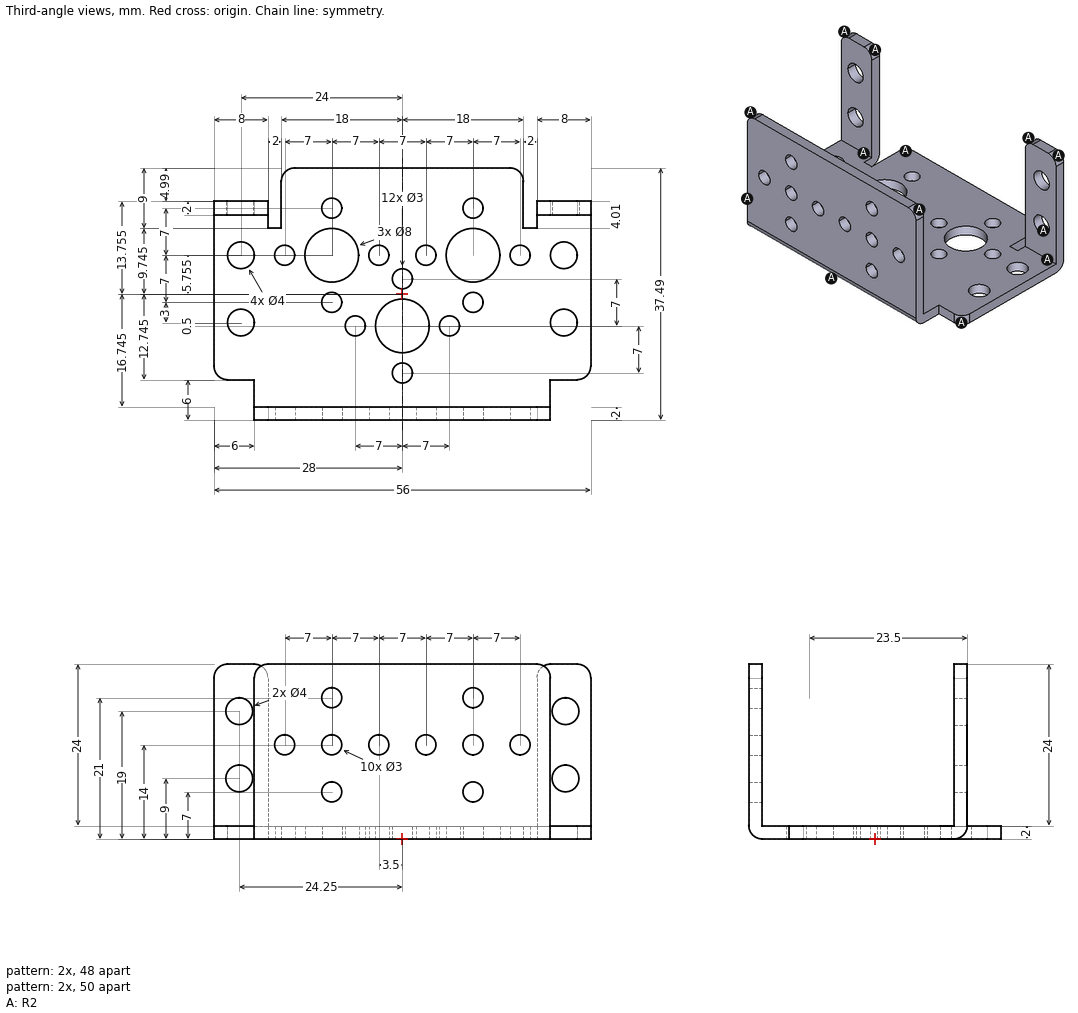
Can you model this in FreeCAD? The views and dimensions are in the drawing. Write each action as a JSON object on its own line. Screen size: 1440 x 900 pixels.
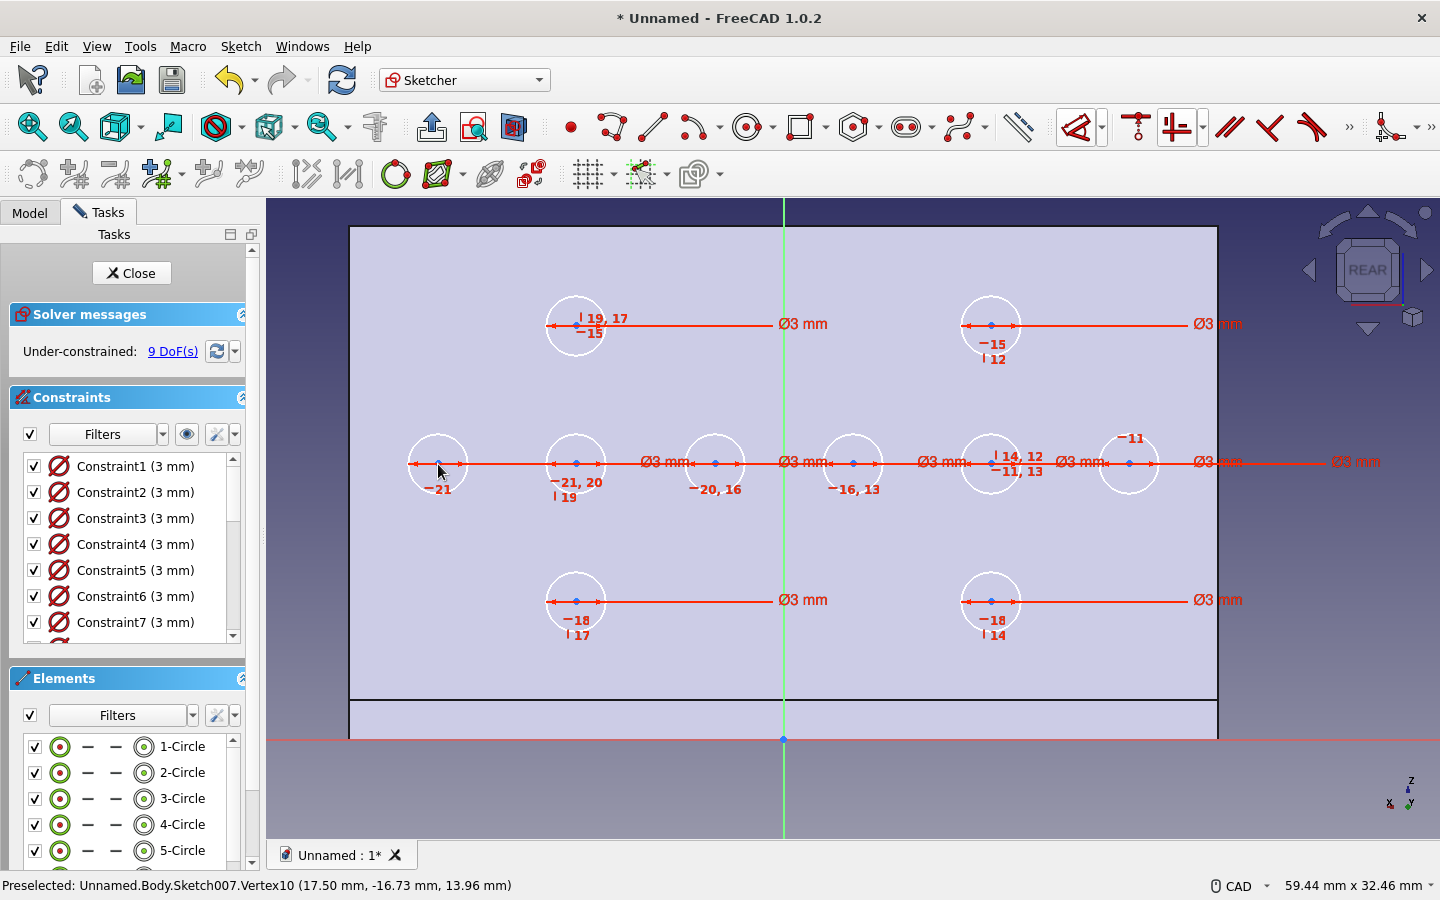
{"action": "left_click", "coordinate": [991, 602]}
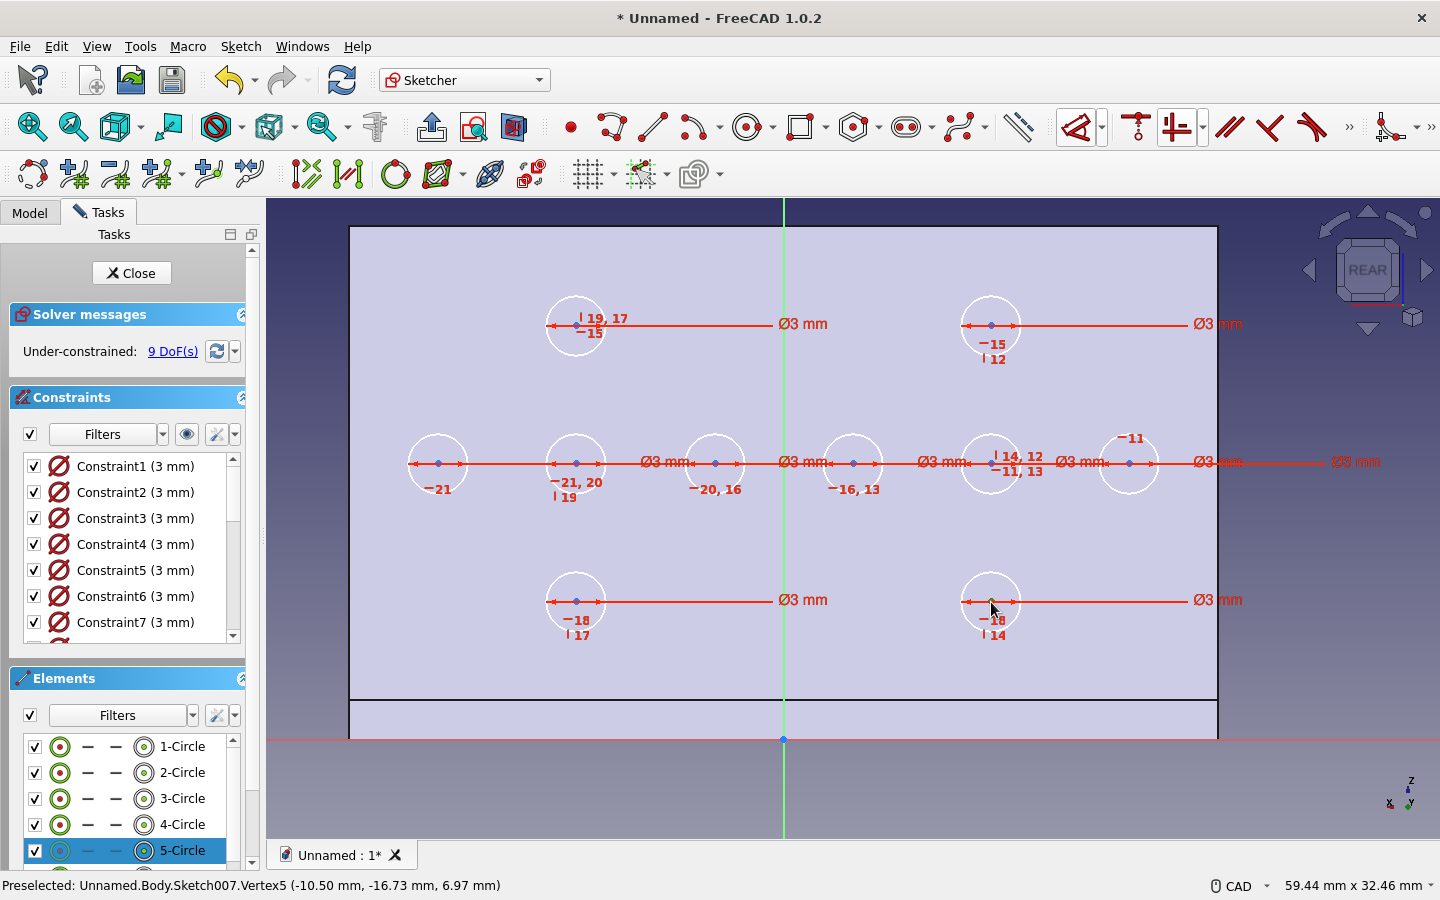
{"action": "key", "text": "i"}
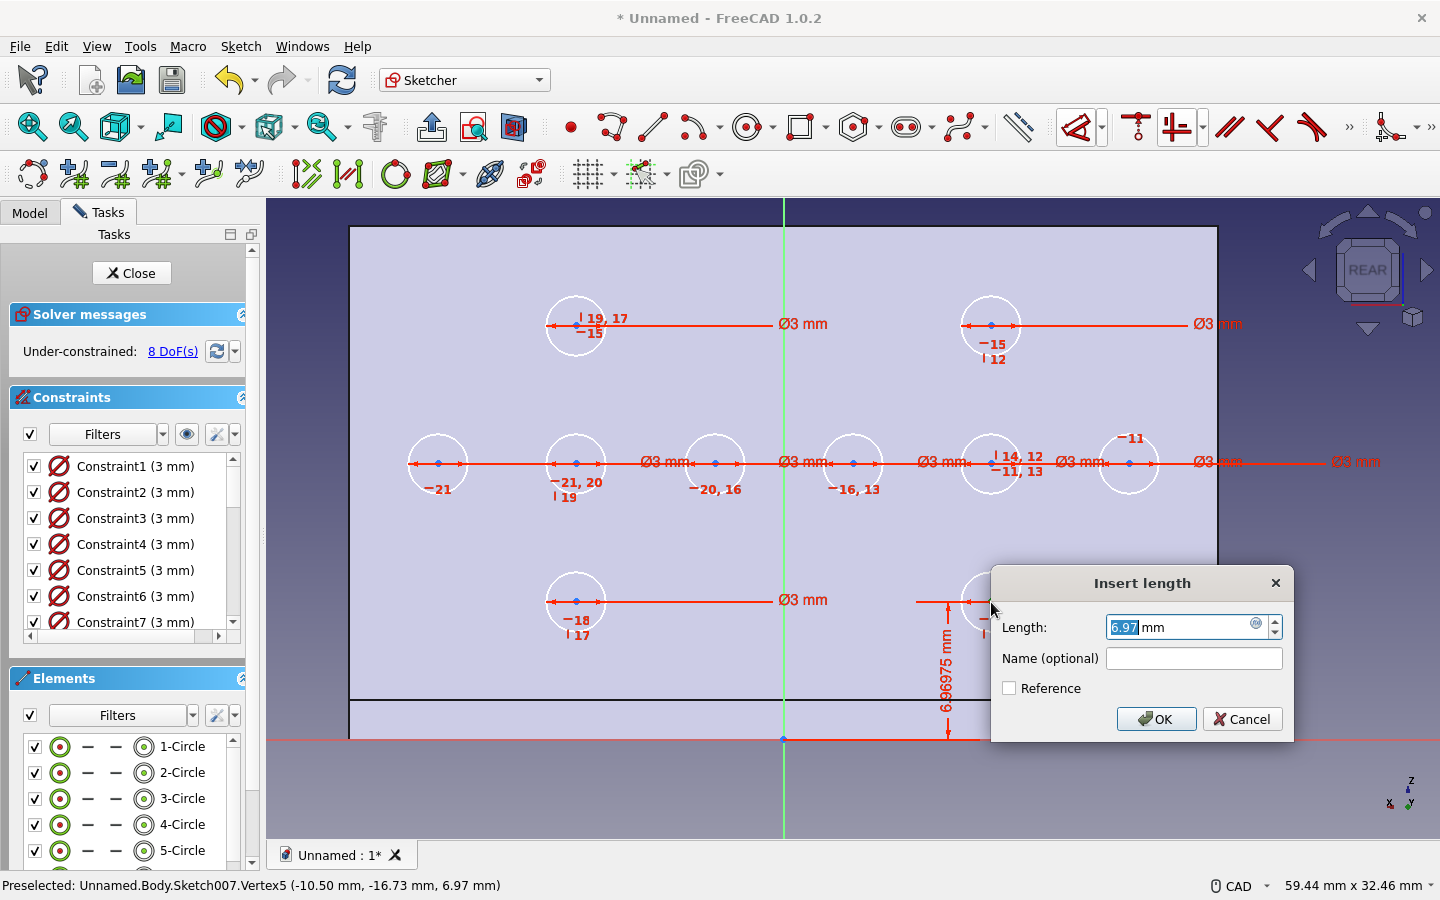
{"action": "type", "text": "7"}
{"action": "key", "text": "Return"}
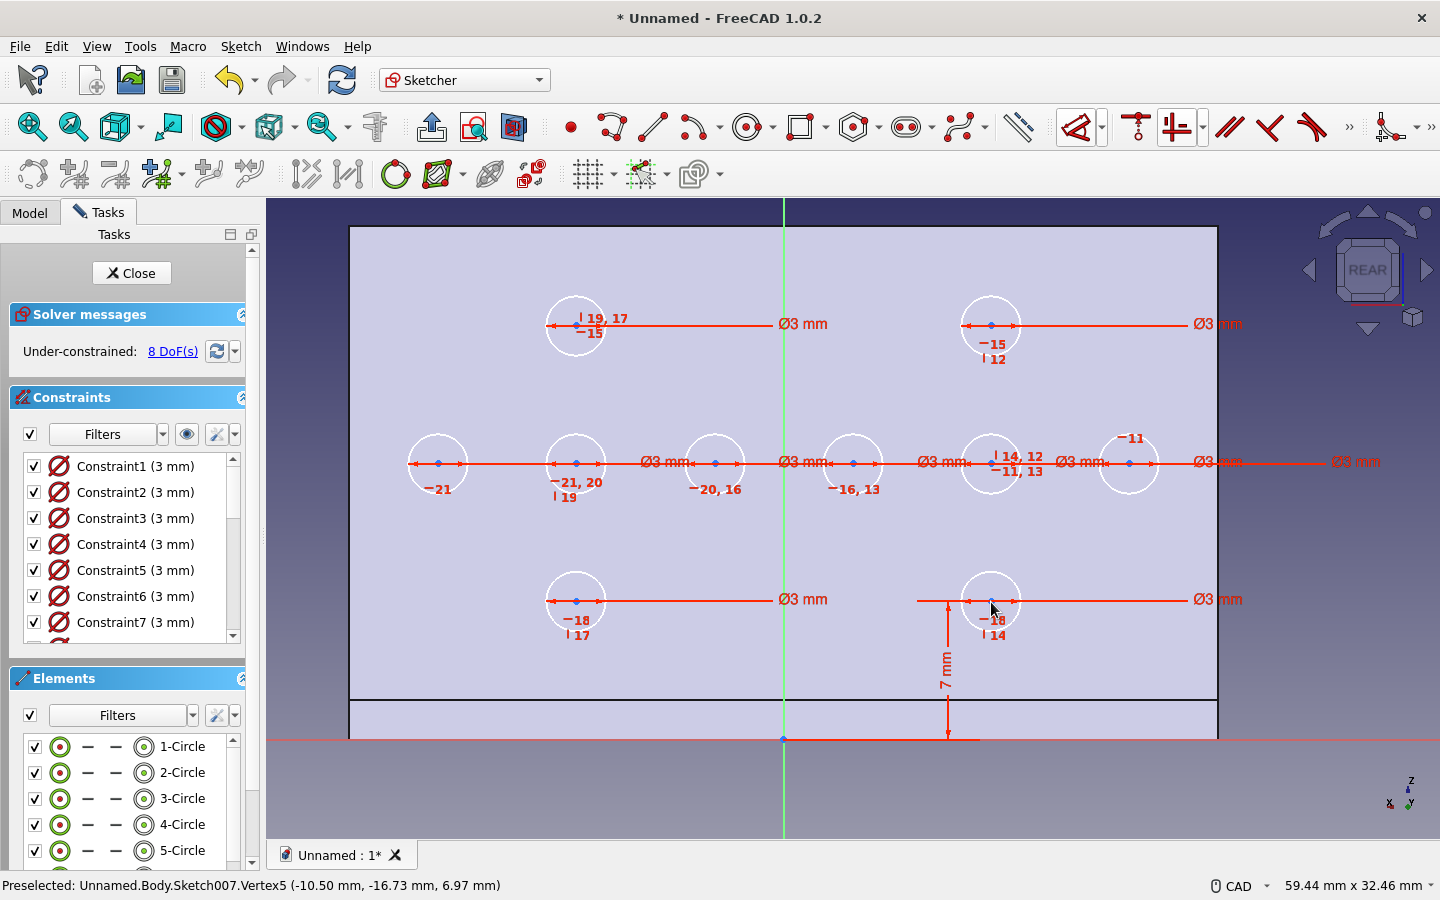
{"action": "left_click", "coordinate": [991, 464]}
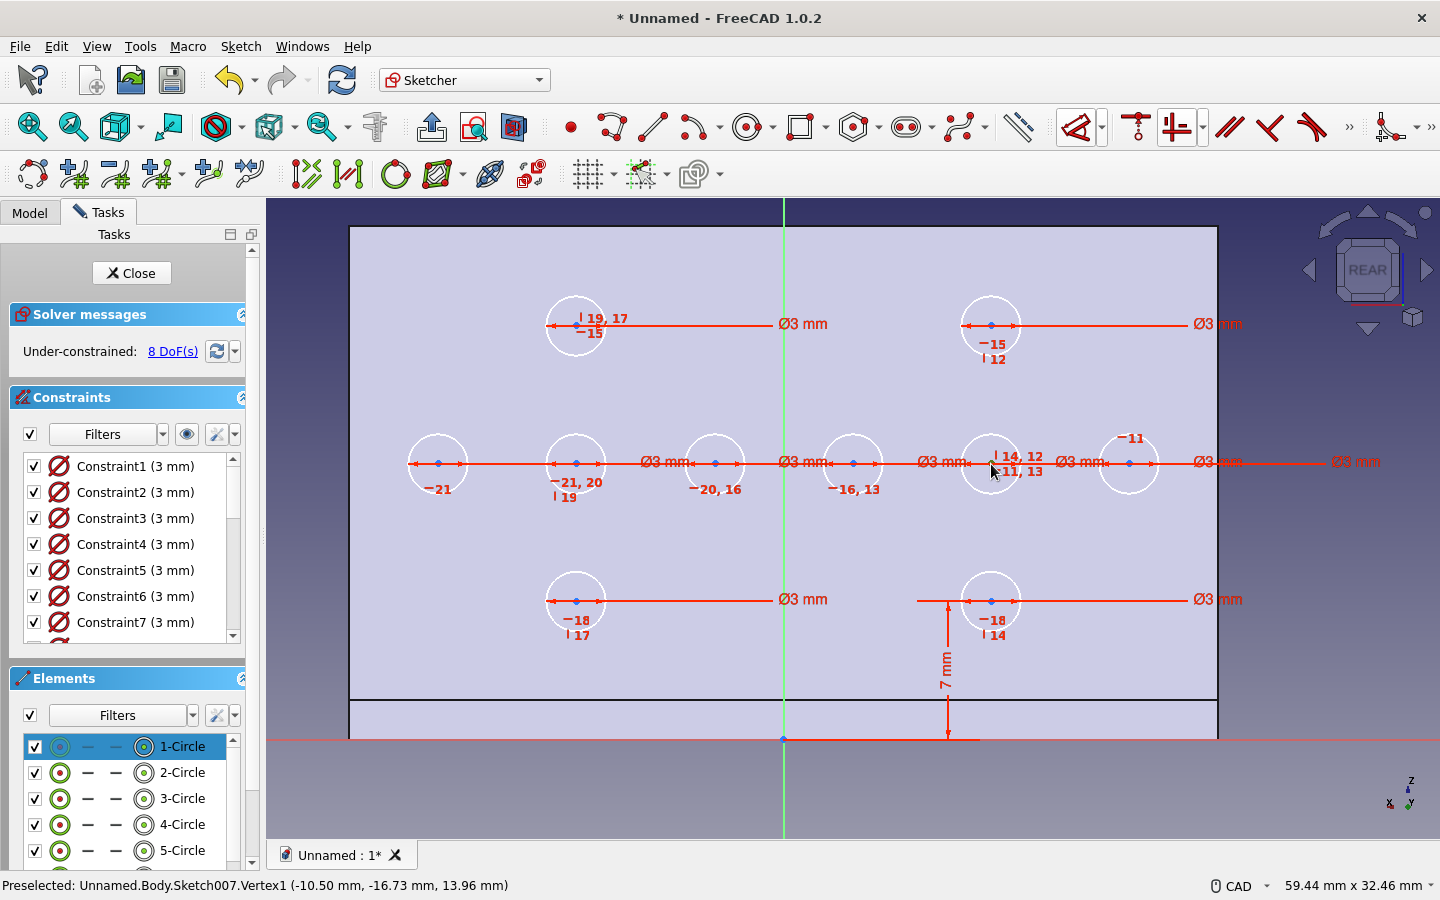
{"action": "key", "text": "i"}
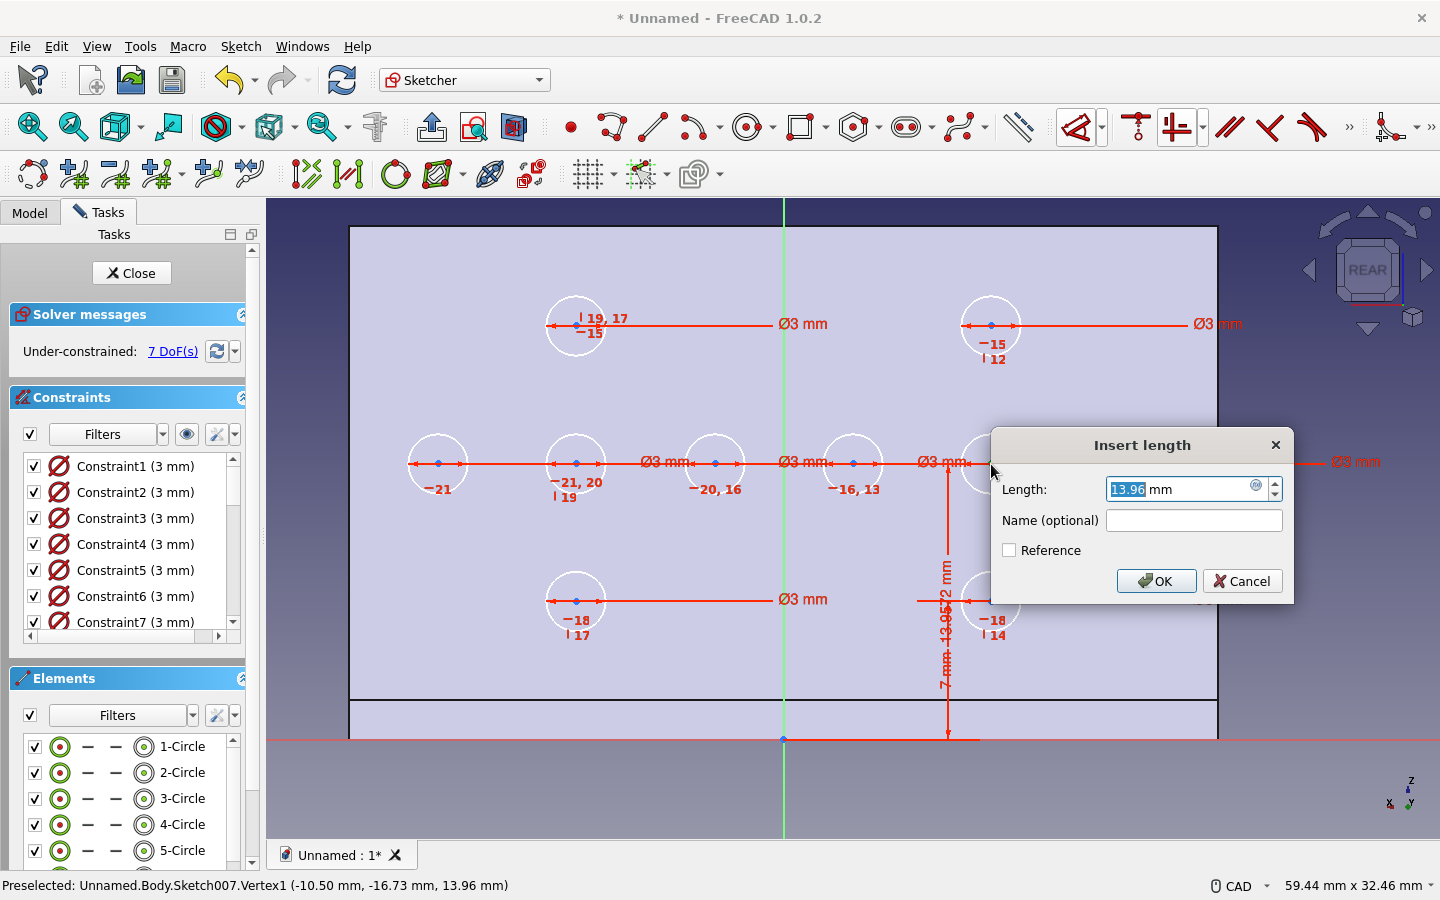
{"action": "type", "text": "14"}
{"action": "key", "text": "Return"}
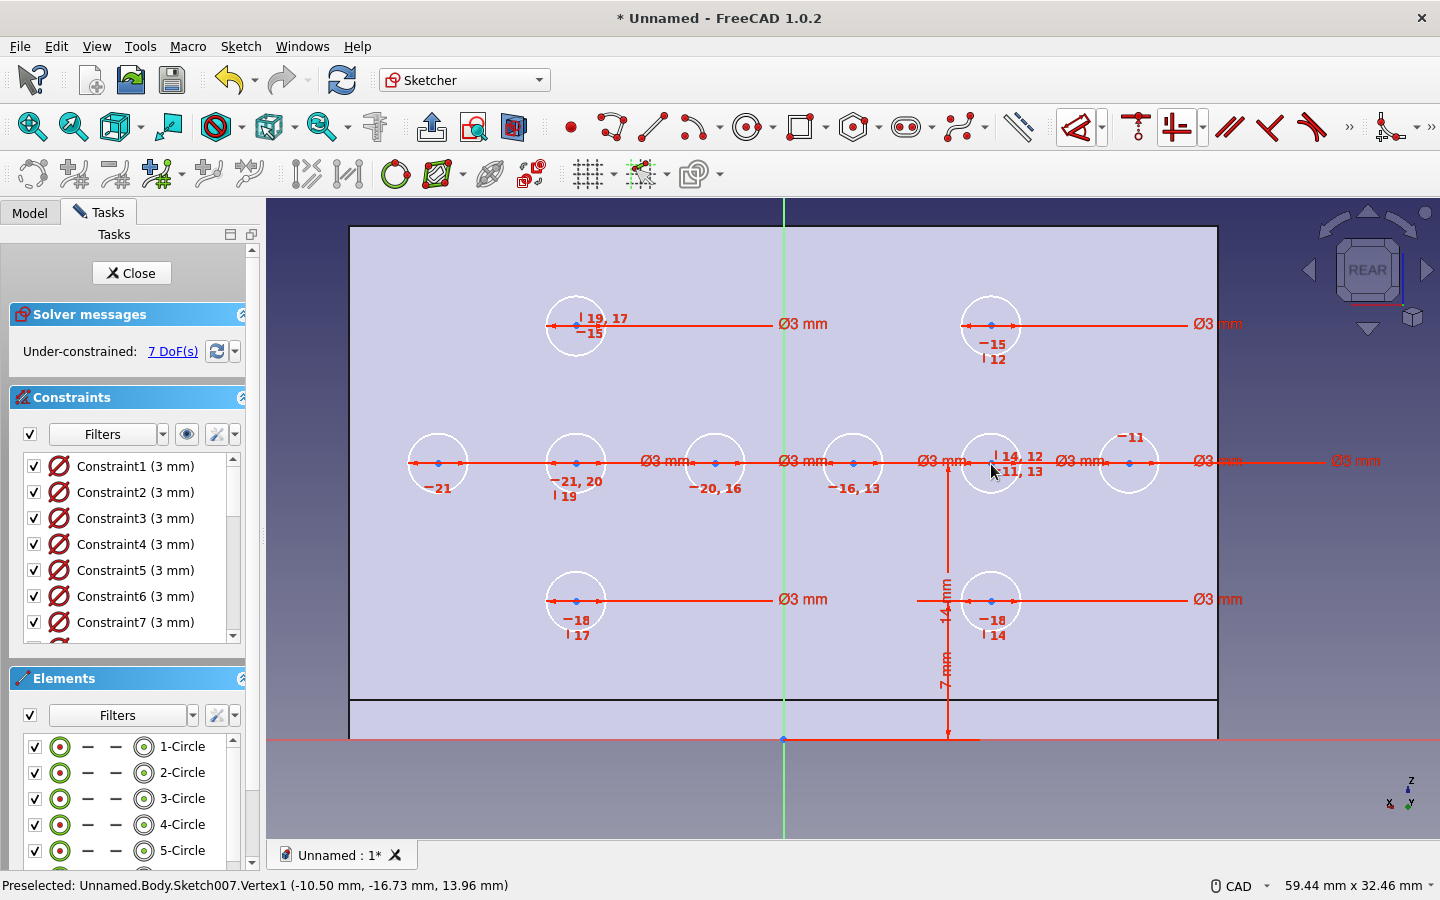
{"action": "left_click", "coordinate": [991, 326]}